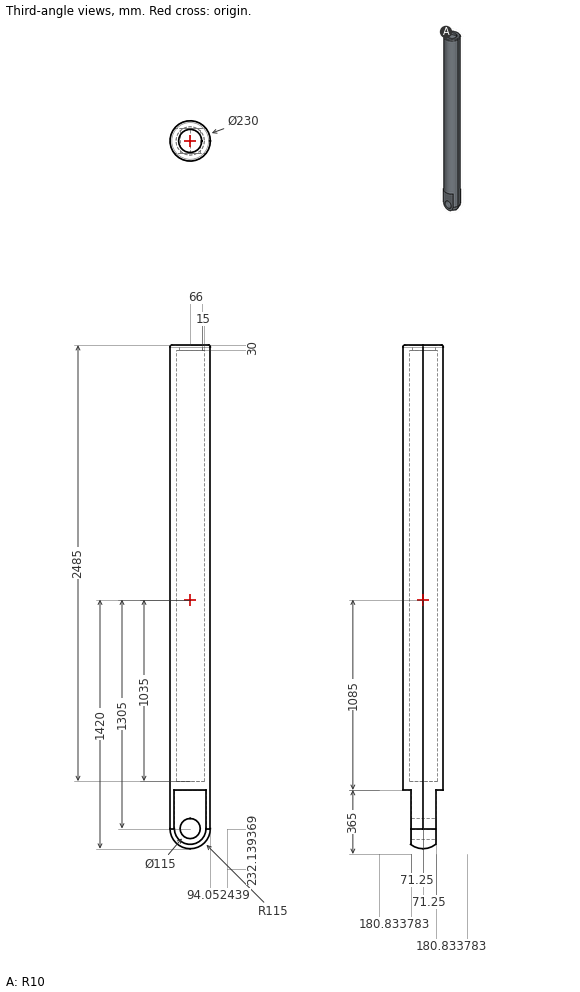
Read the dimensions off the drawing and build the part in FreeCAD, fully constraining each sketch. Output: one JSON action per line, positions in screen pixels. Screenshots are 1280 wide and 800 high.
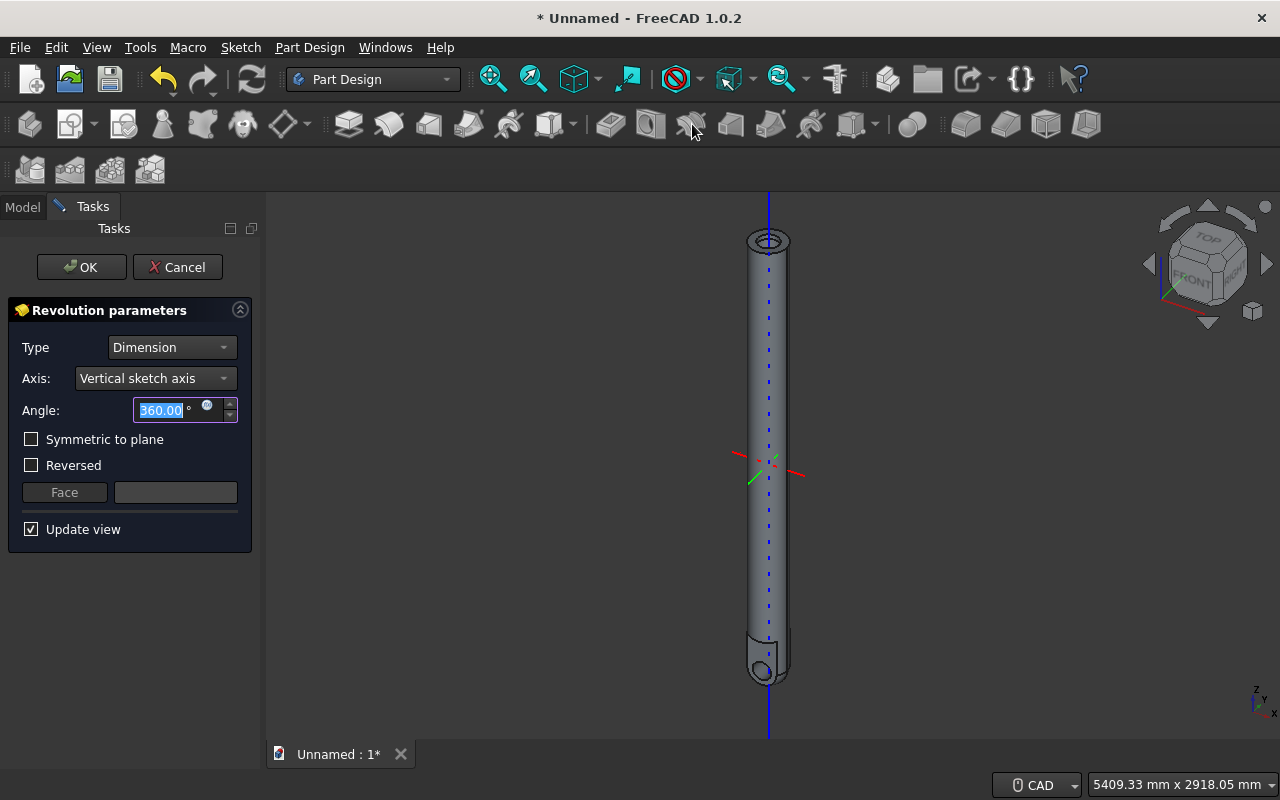
{"action": "left_click", "coordinate": [82, 267]}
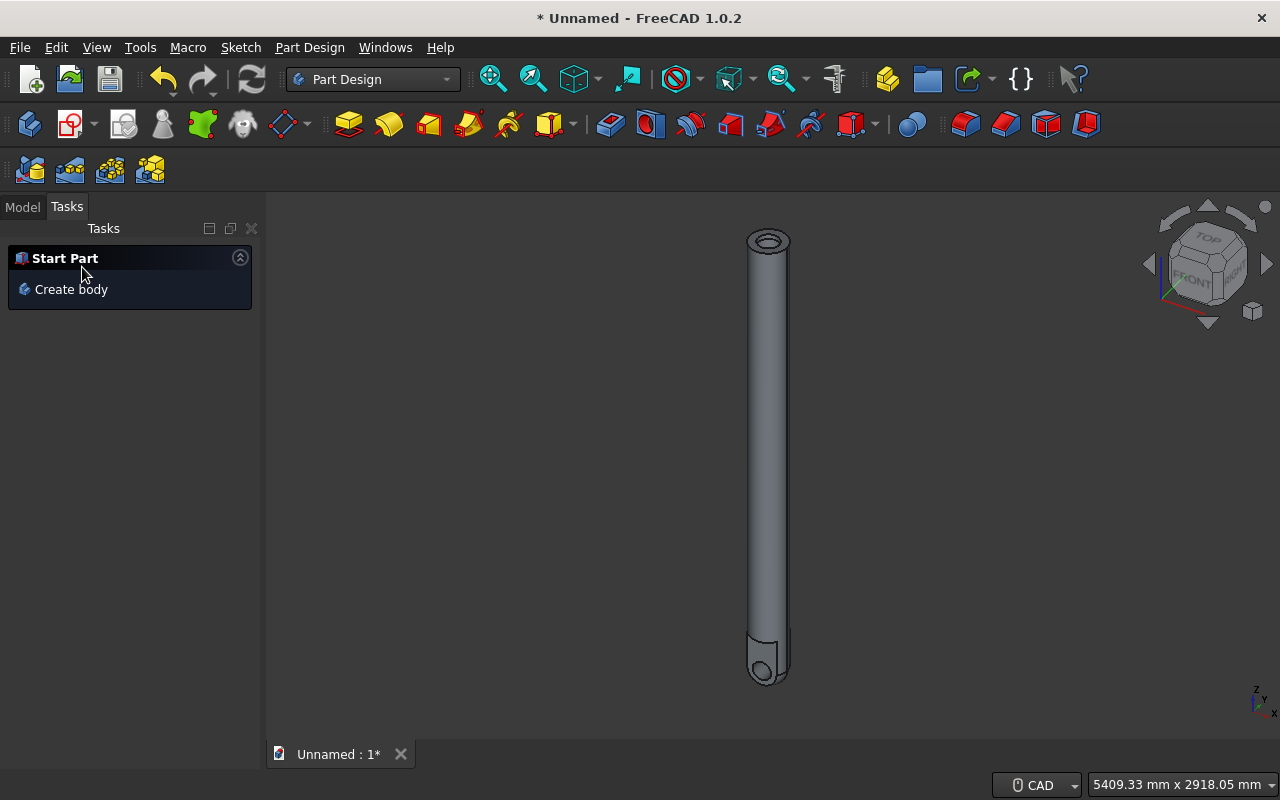
{"action": "left_click", "coordinate": [747, 242]}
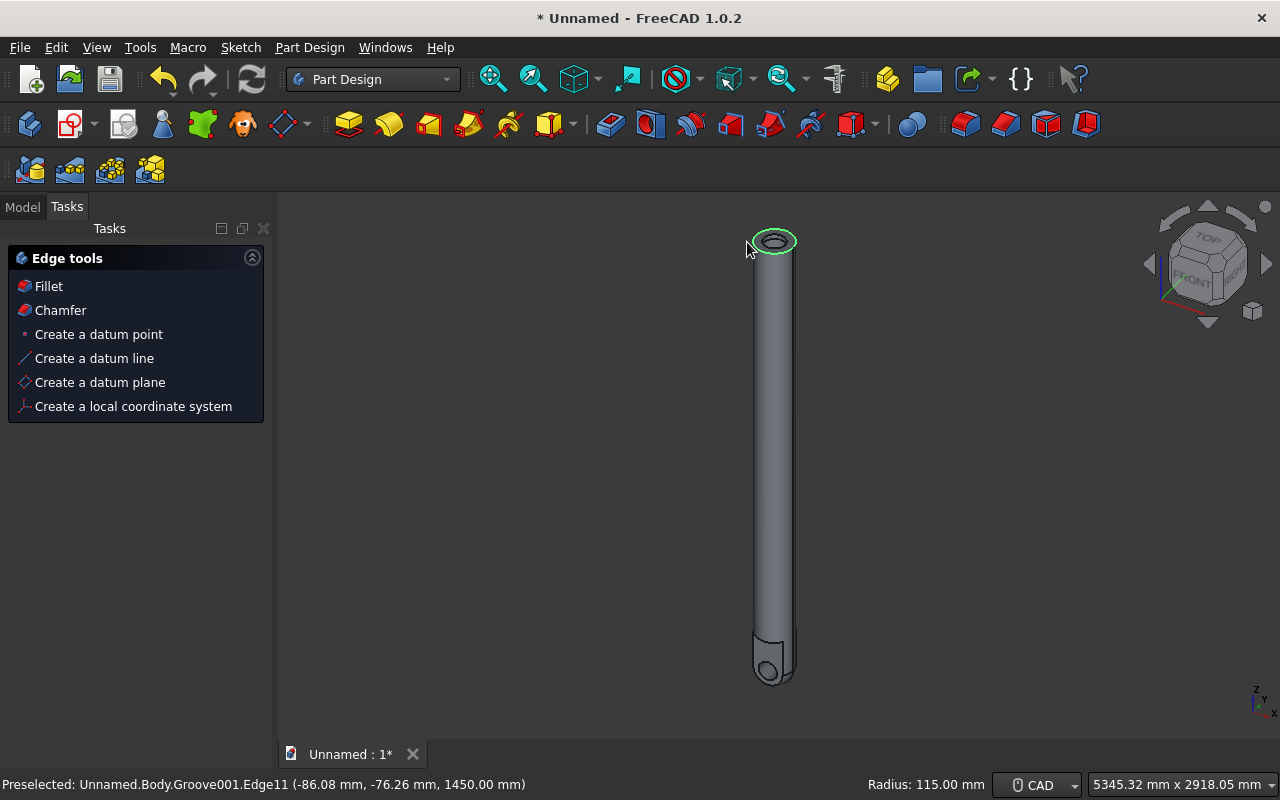
{"action": "left_click", "coordinate": [966, 124]}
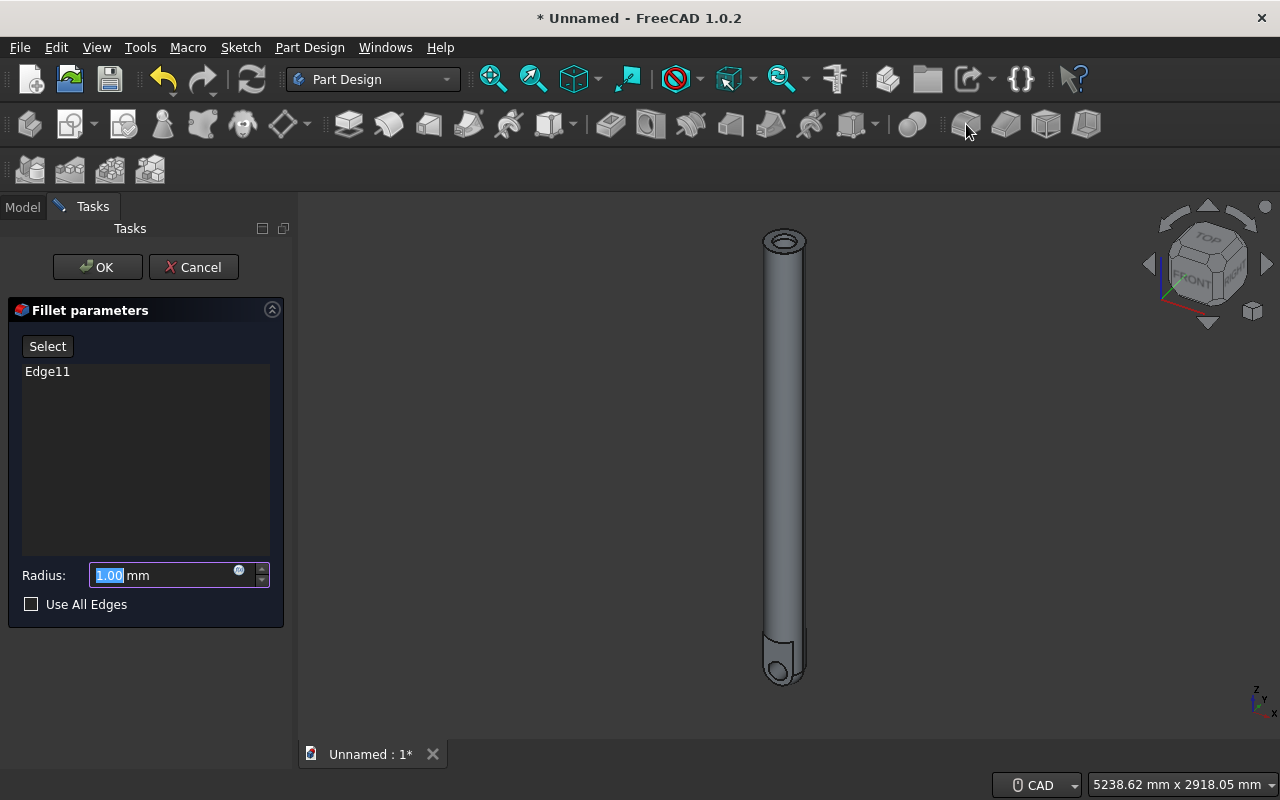
{"action": "type", "text": "10"}
{"action": "key", "text": "Tab"}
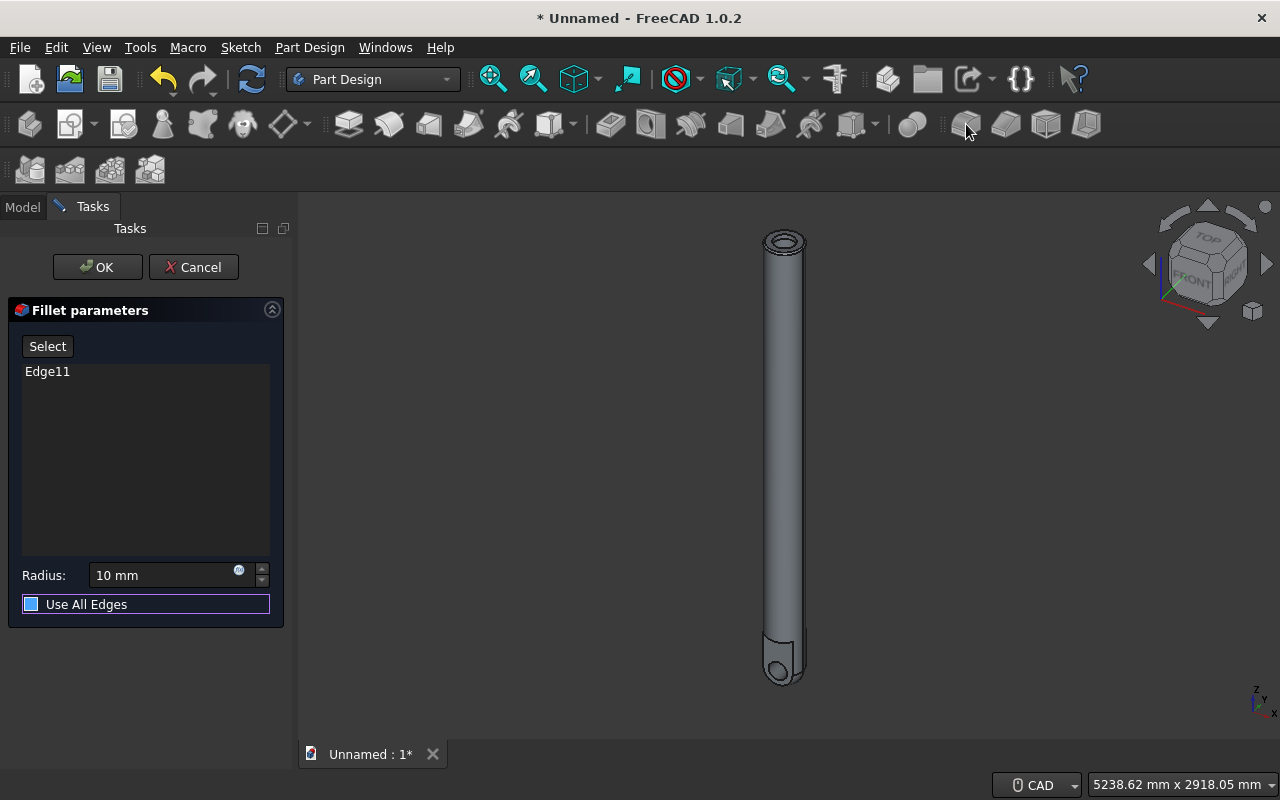
{"action": "left_click", "coordinate": [98, 267]}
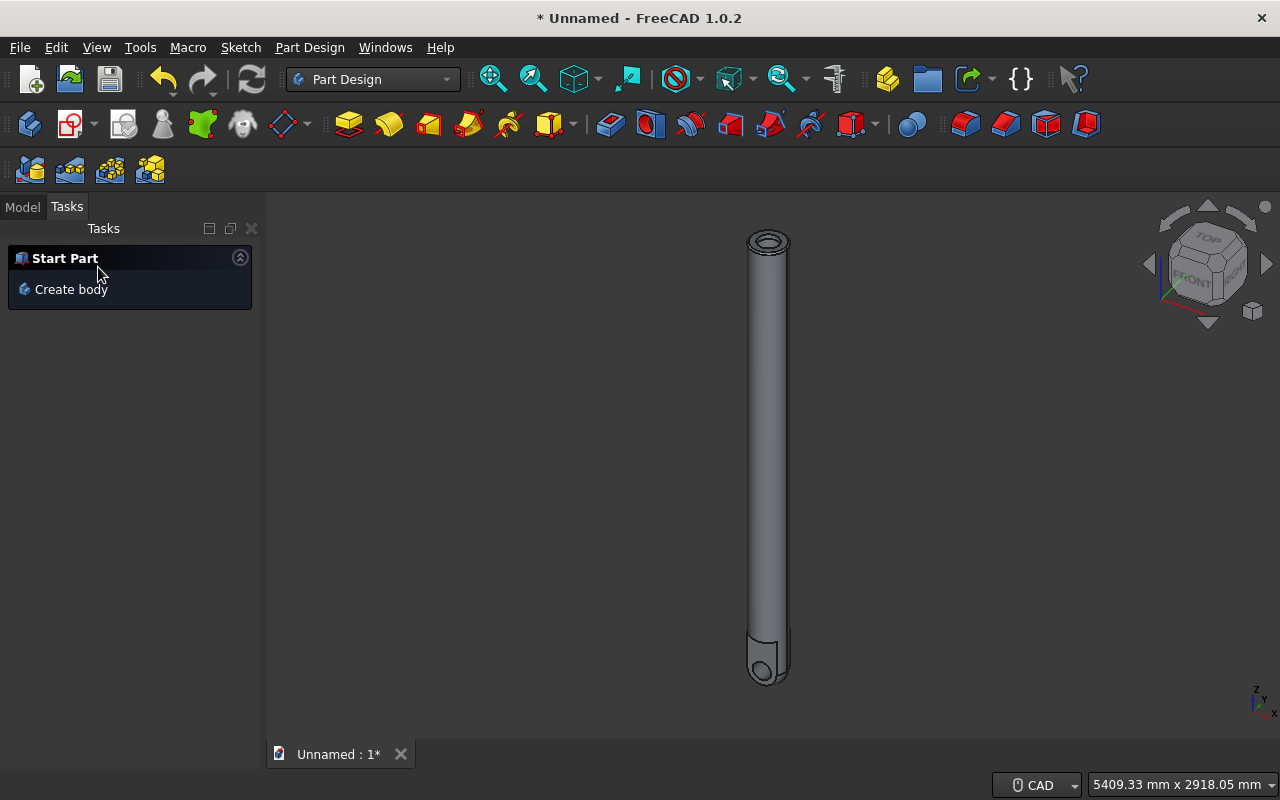
{"action": "key", "text": "0"}